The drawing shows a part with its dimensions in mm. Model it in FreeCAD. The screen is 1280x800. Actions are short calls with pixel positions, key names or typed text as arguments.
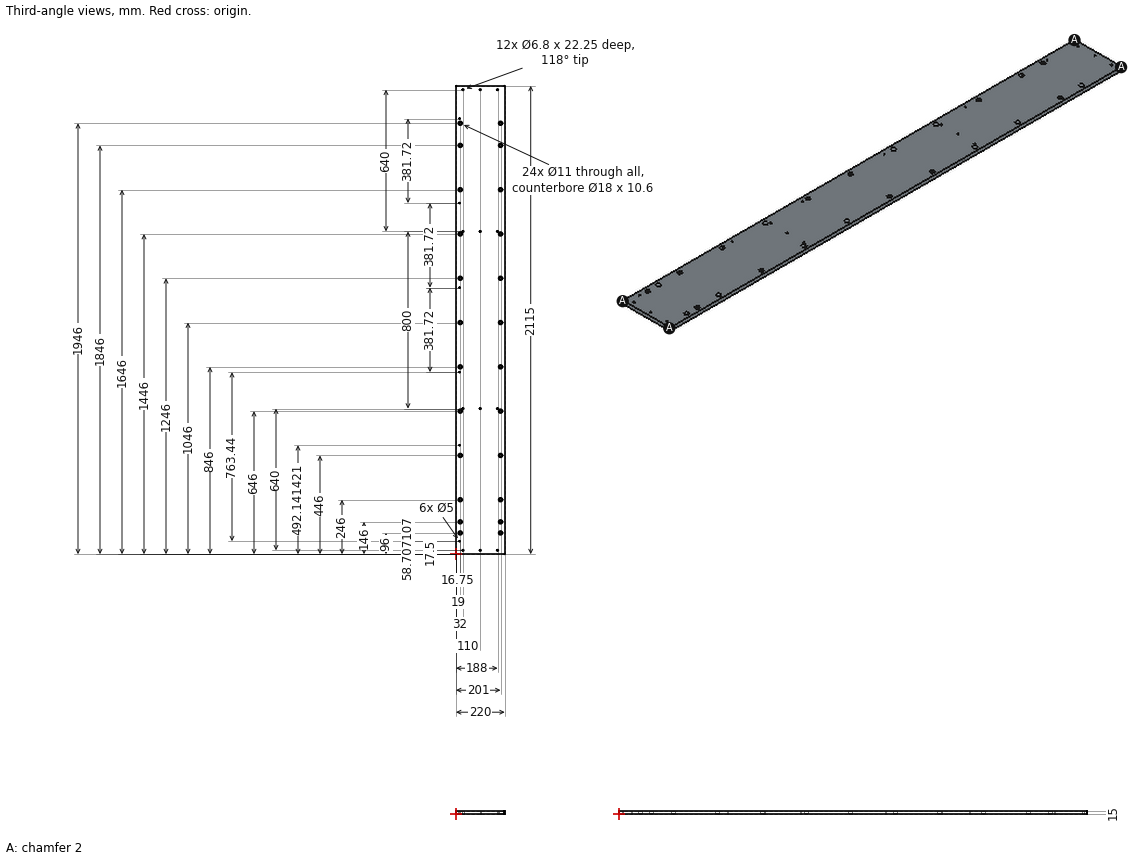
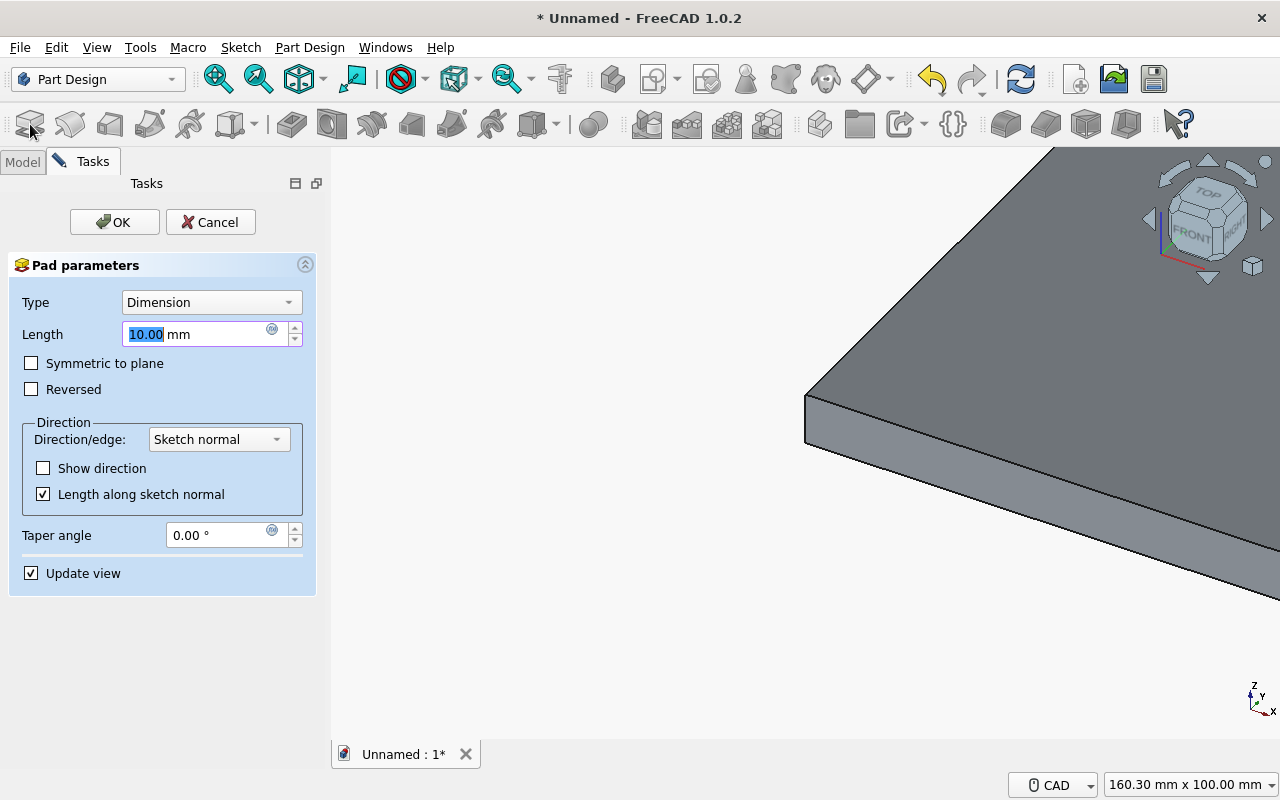
text(15)
key(Tab)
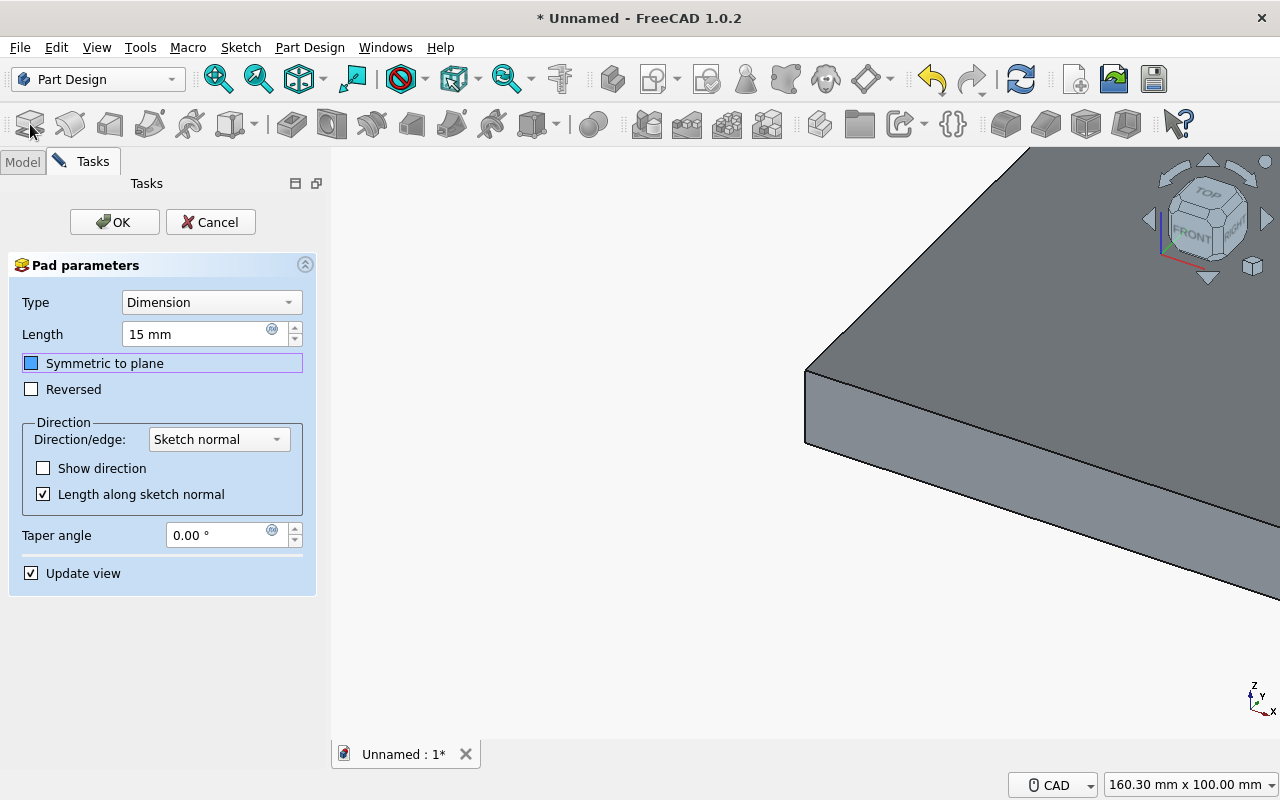
click(115, 222)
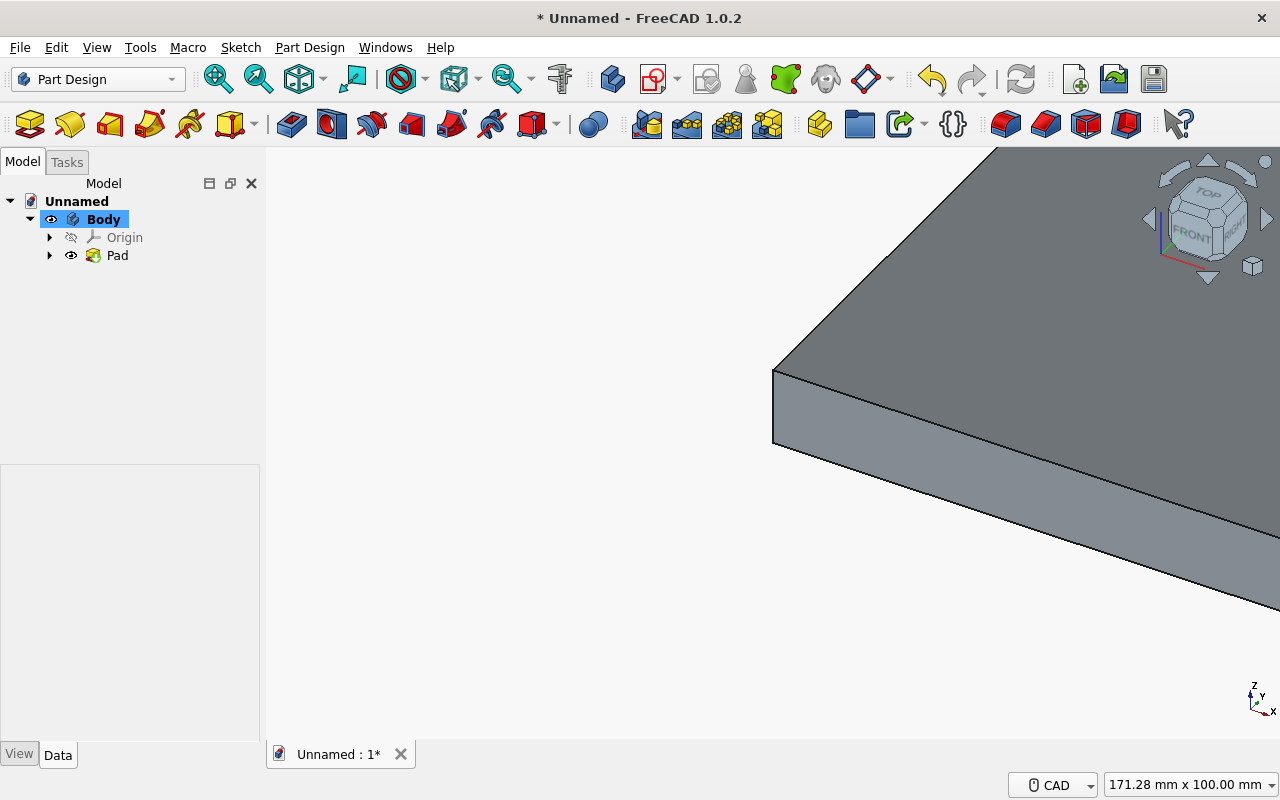
click(220, 80)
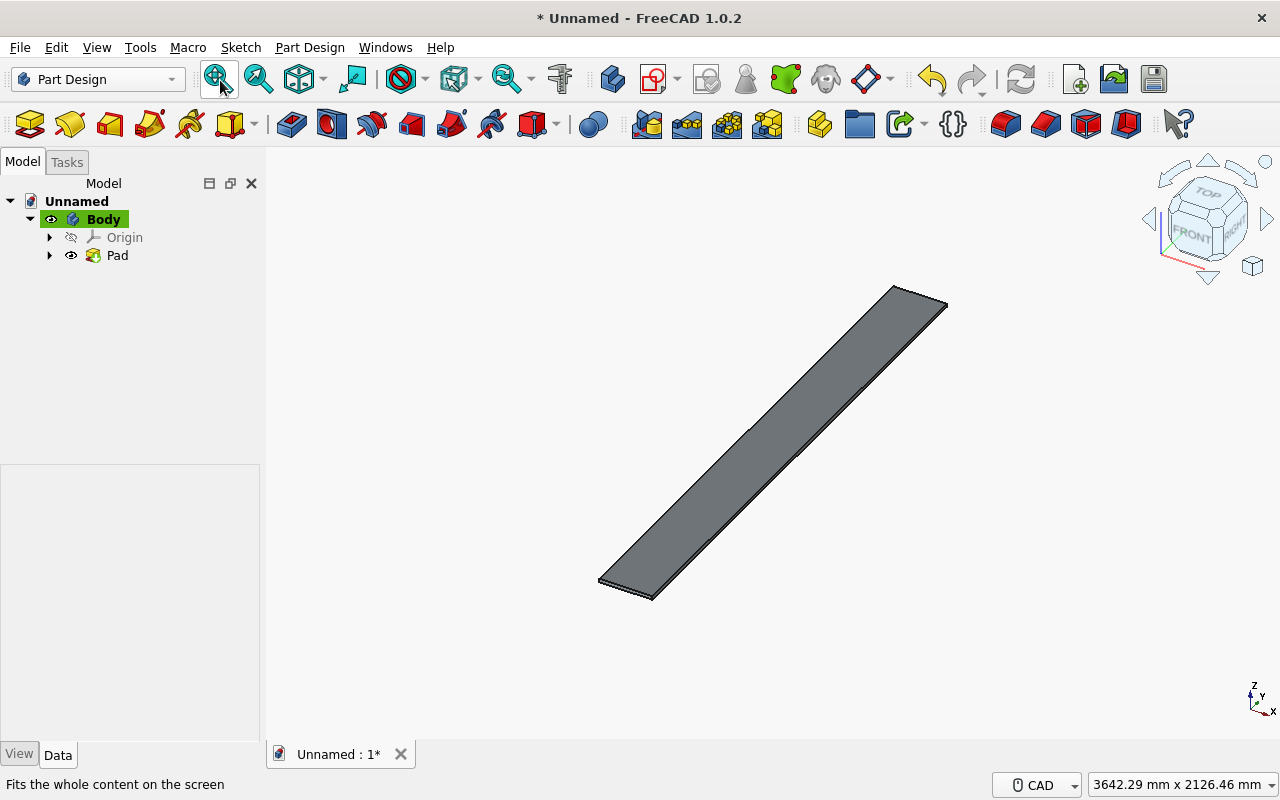
scroll(652, 597, up, 12)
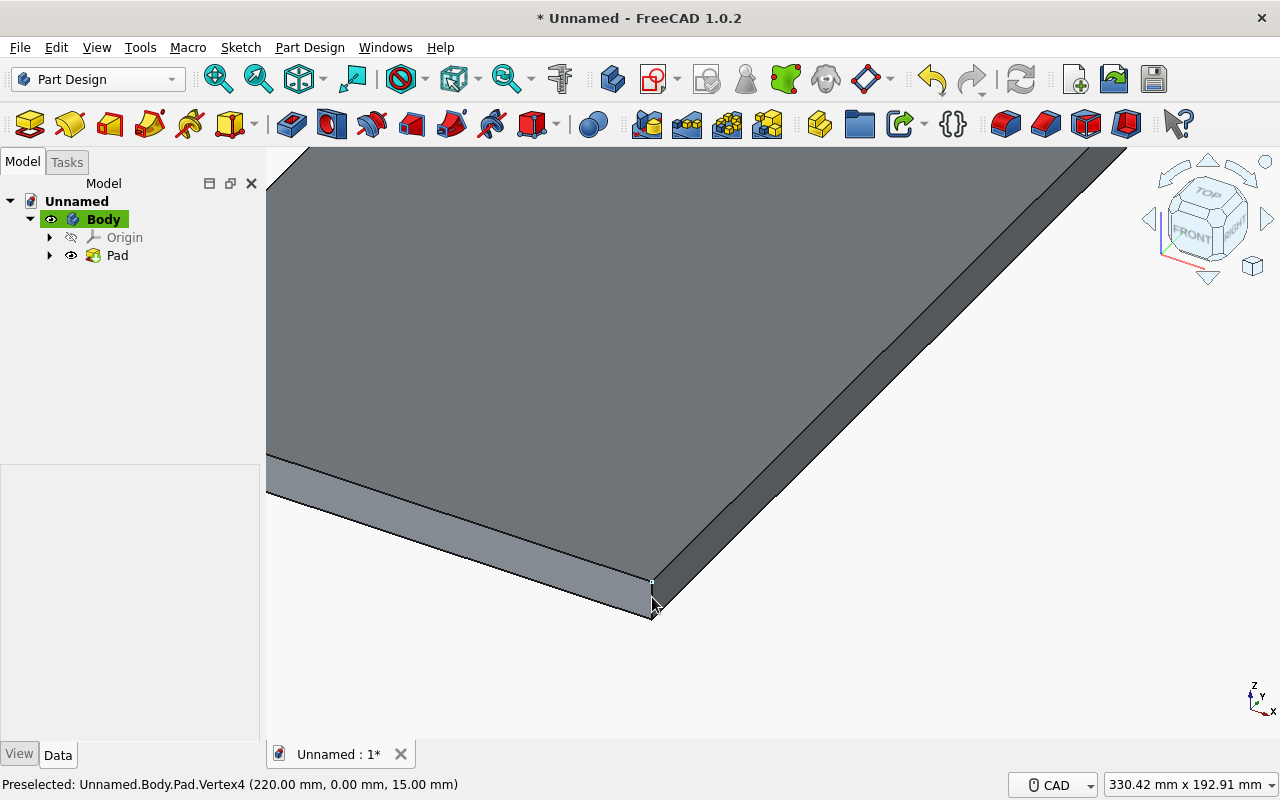
click(652, 600)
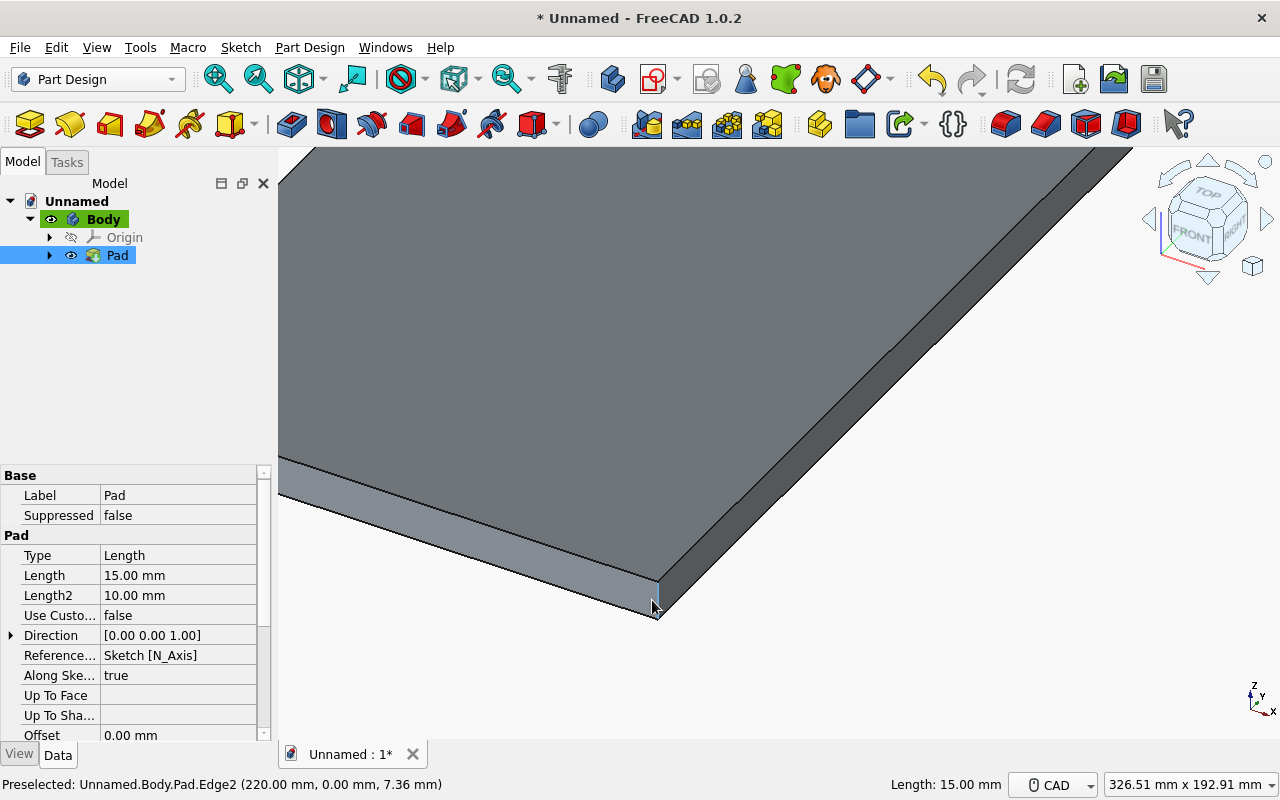
click(220, 80)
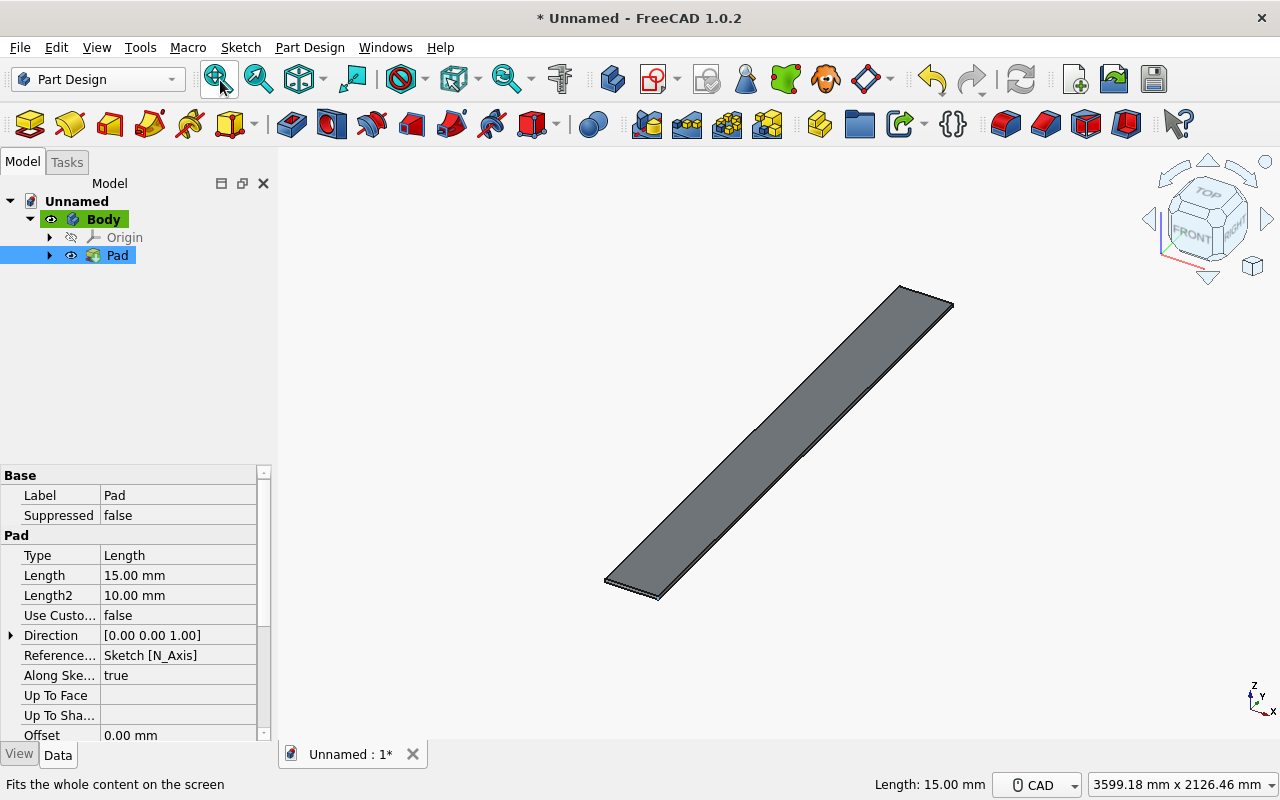
key(0)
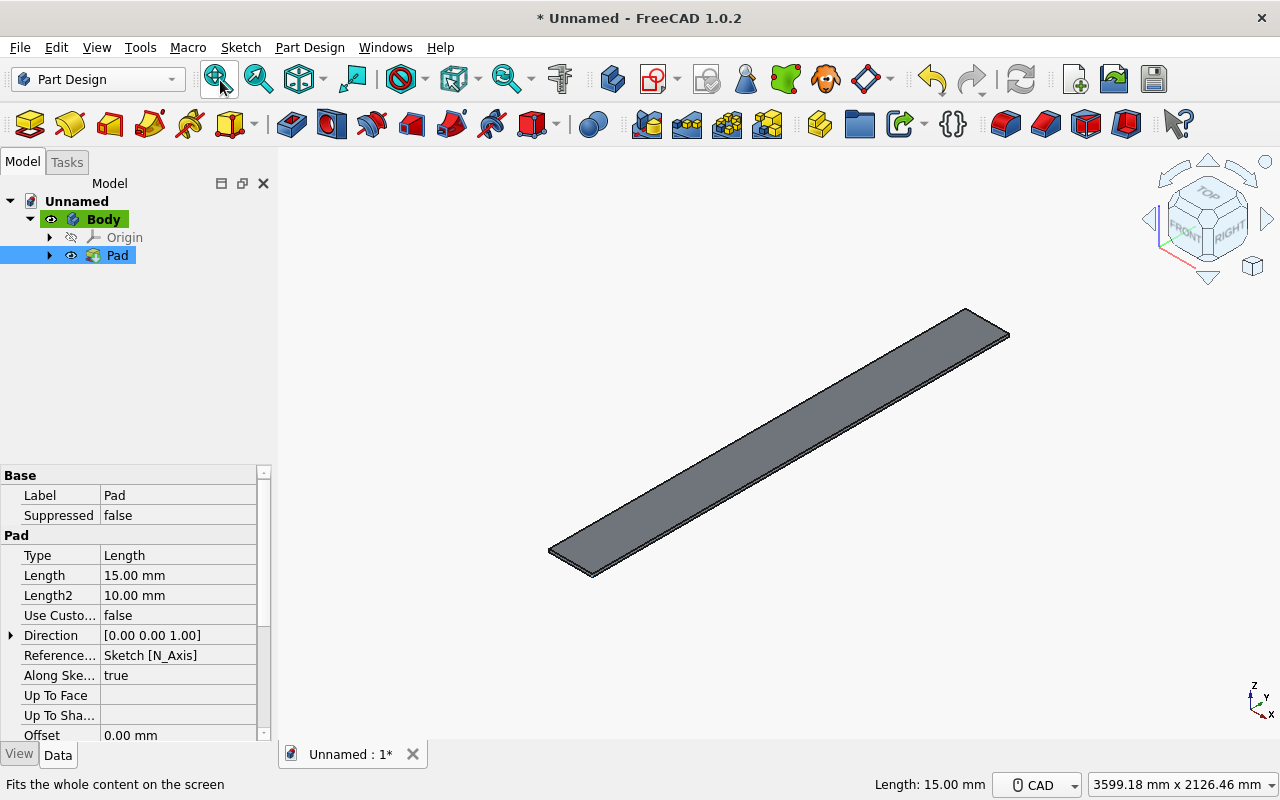
scroll(549, 550, up, 12)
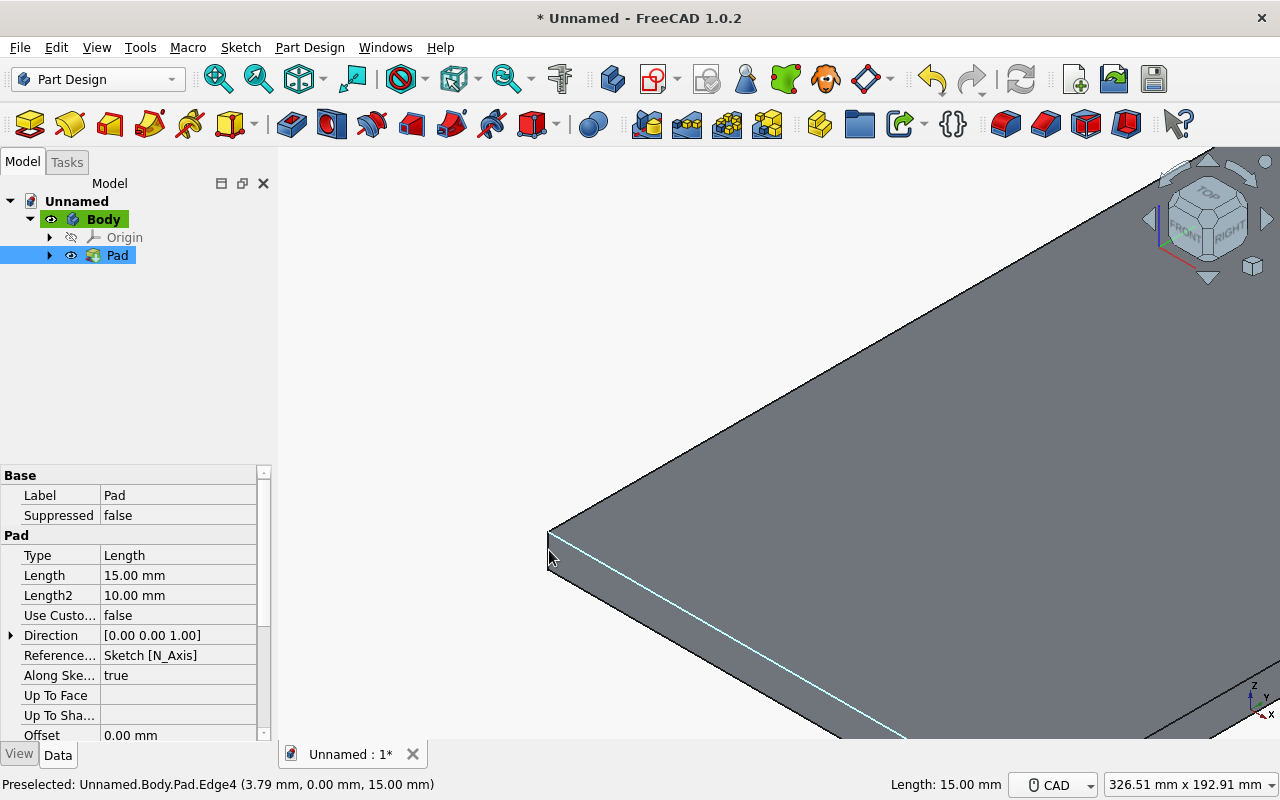
click(220, 80)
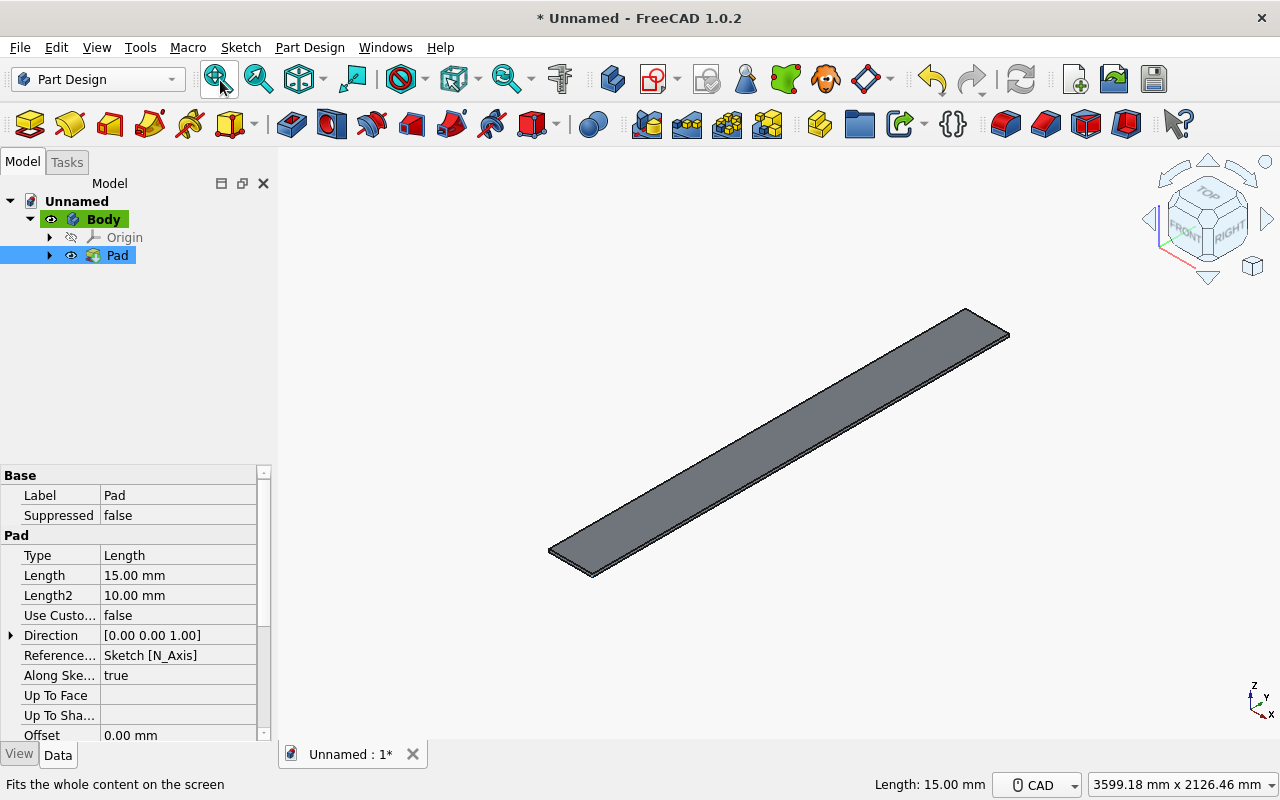
key(2)